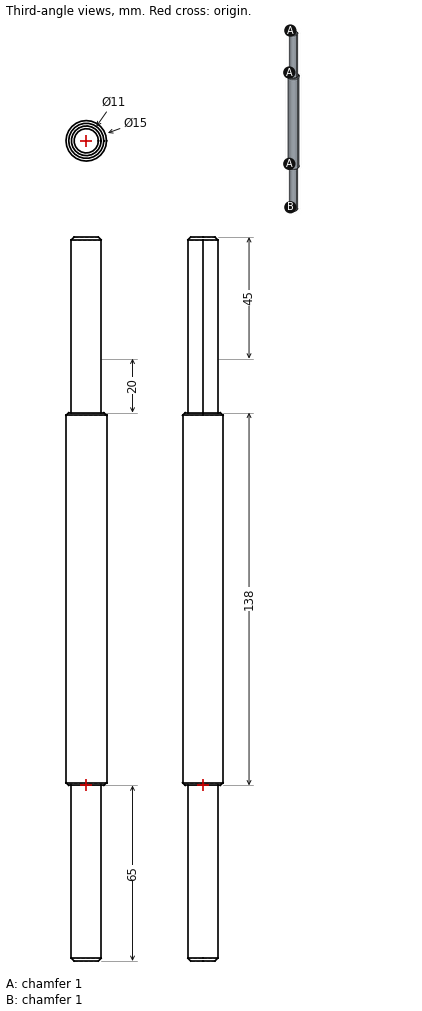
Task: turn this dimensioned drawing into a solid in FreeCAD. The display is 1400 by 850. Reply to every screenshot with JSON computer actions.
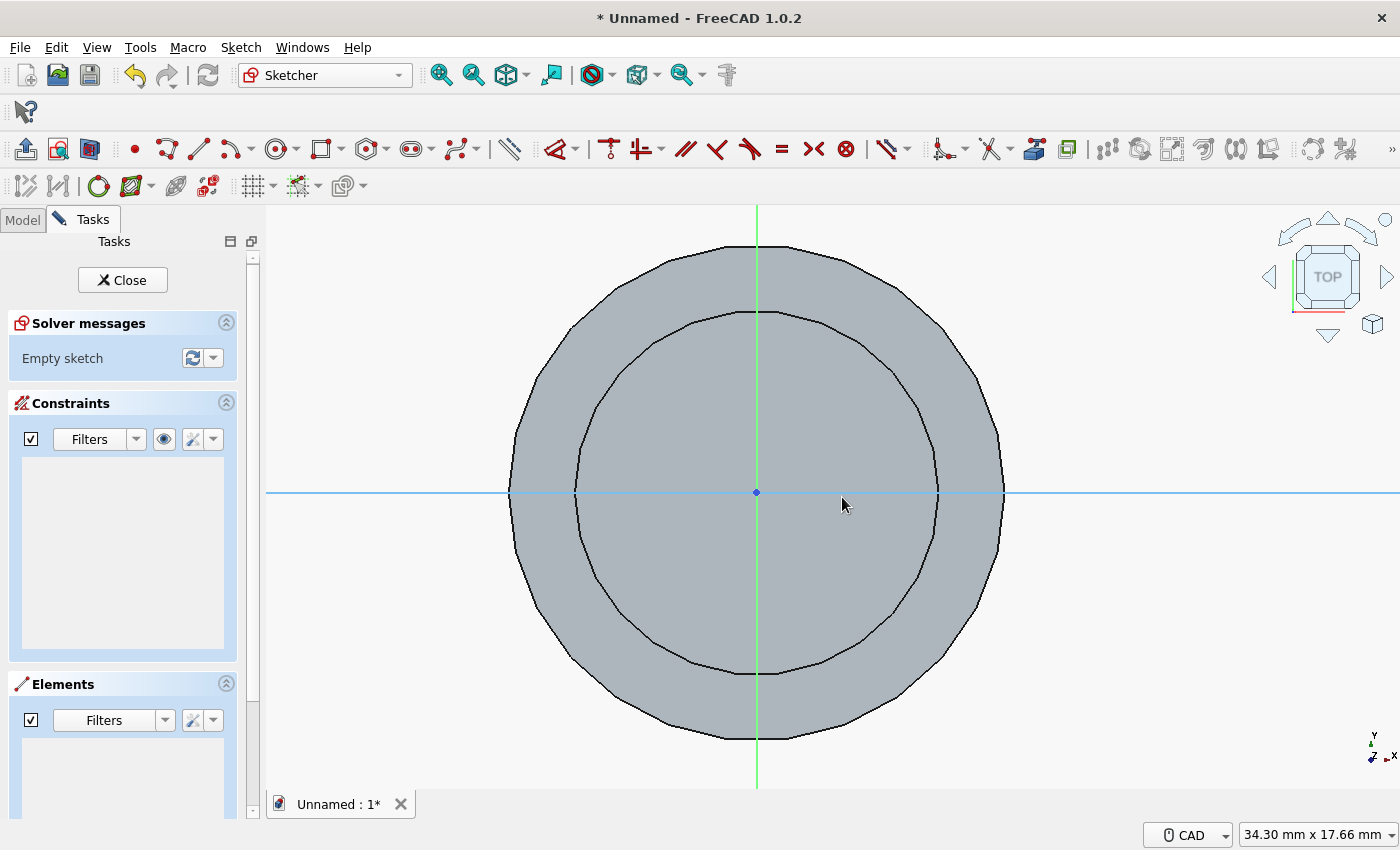
{"action": "left_click", "coordinate": [276, 150]}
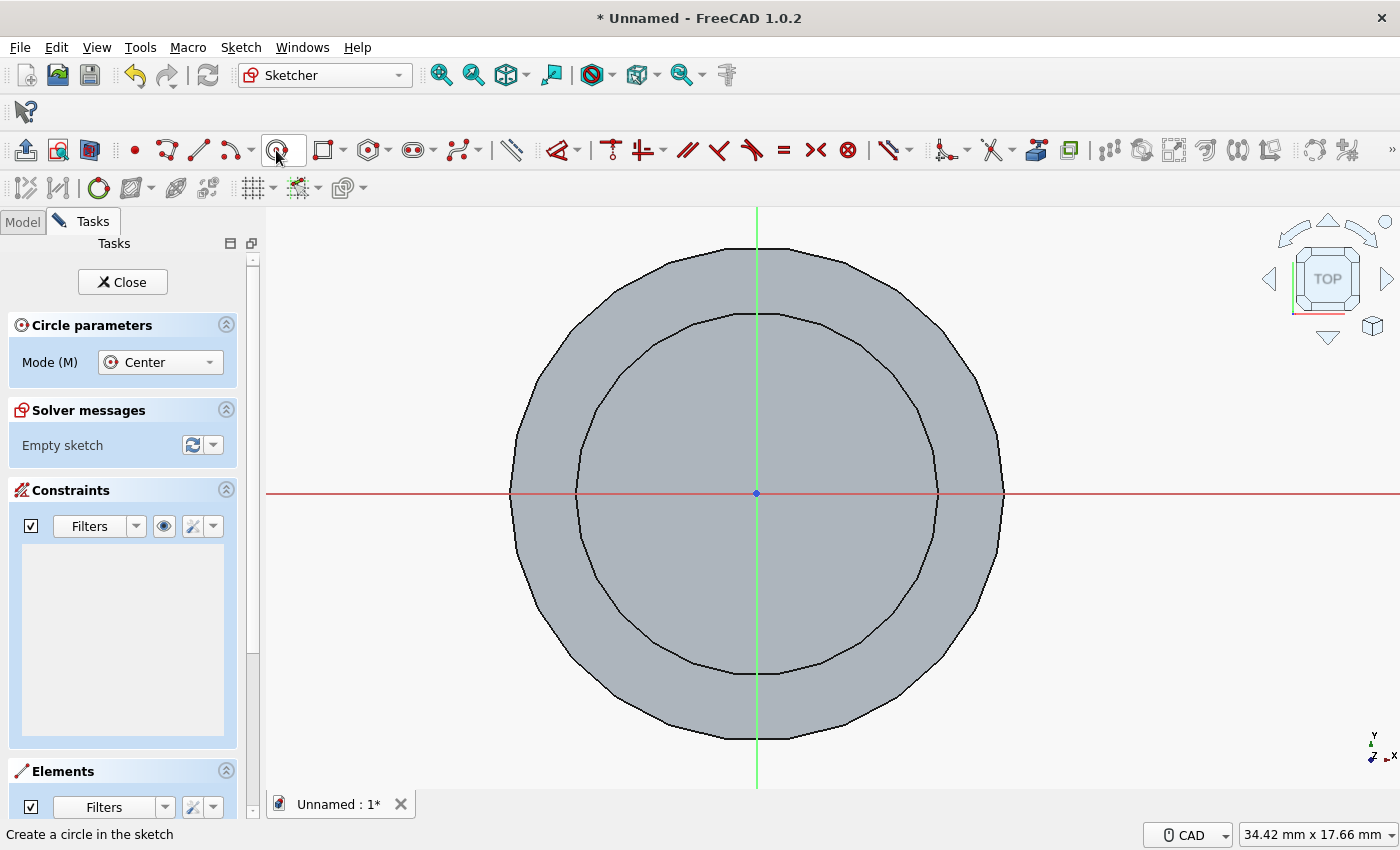
{"action": "left_click", "coordinate": [757, 494]}
{"action": "mouse_move", "coordinate": [885, 366]}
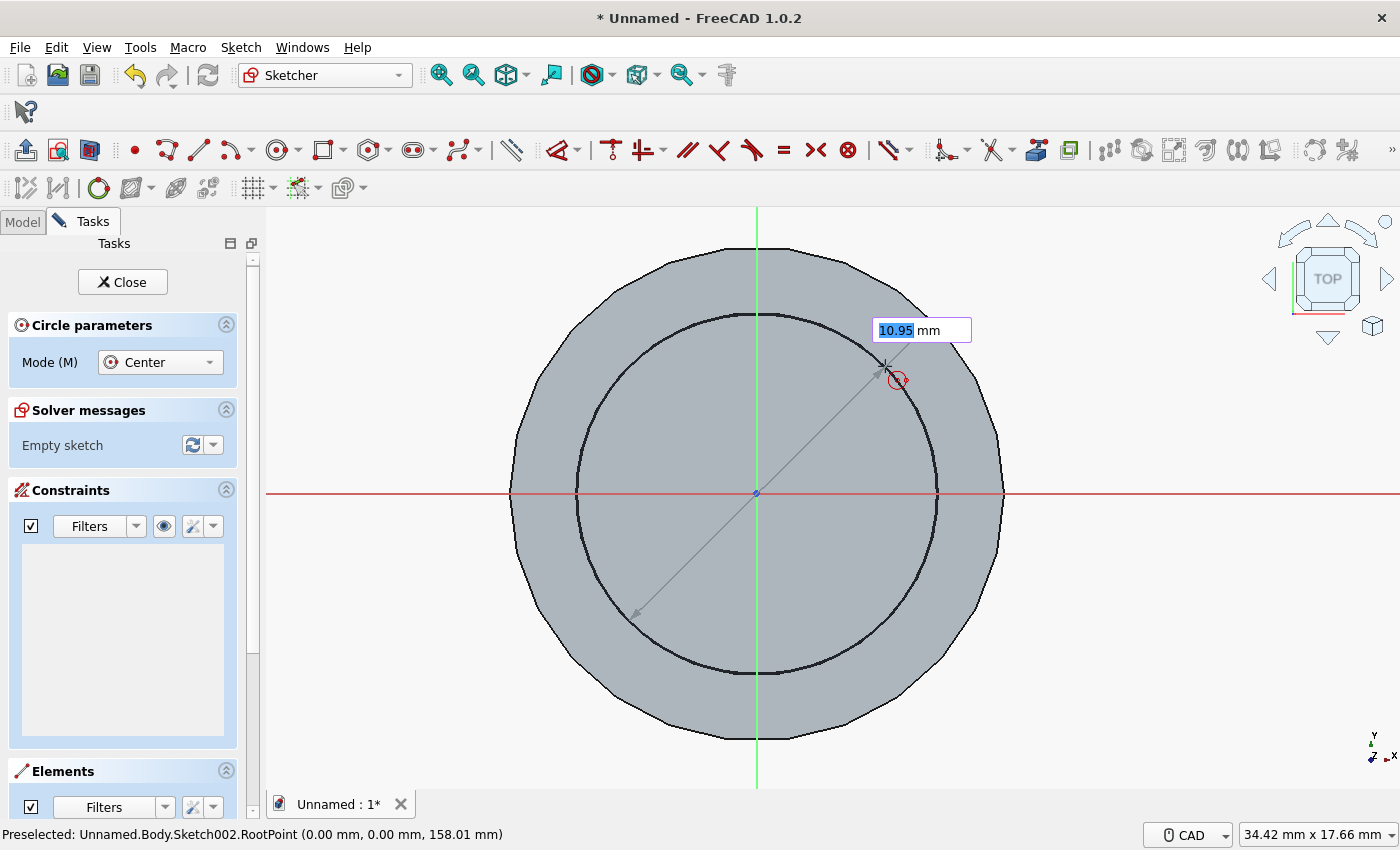
{"action": "type", "text": "11"}
{"action": "key", "text": "Return"}
{"action": "key", "text": "Escape"}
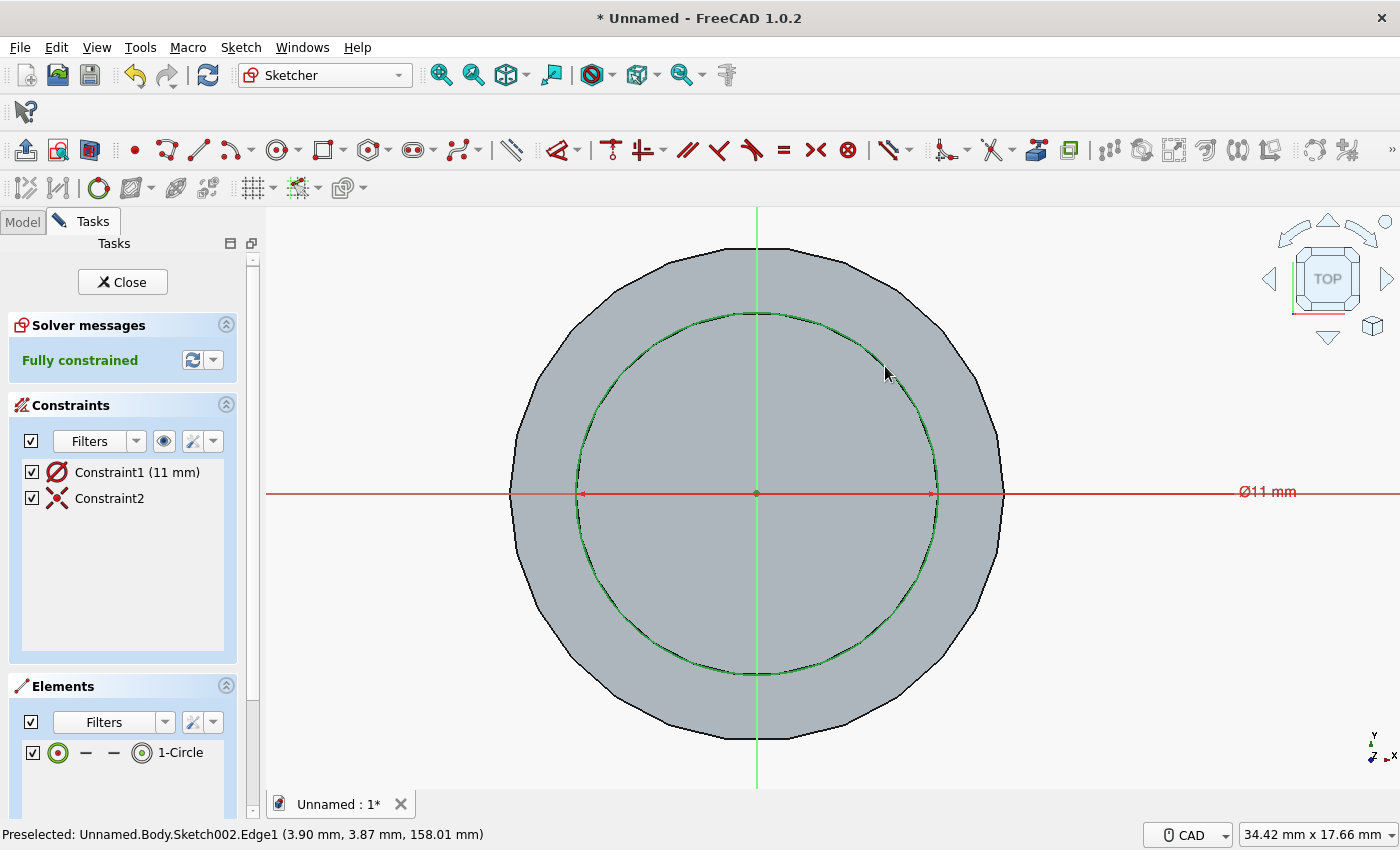
{"action": "left_click", "coordinate": [123, 282]}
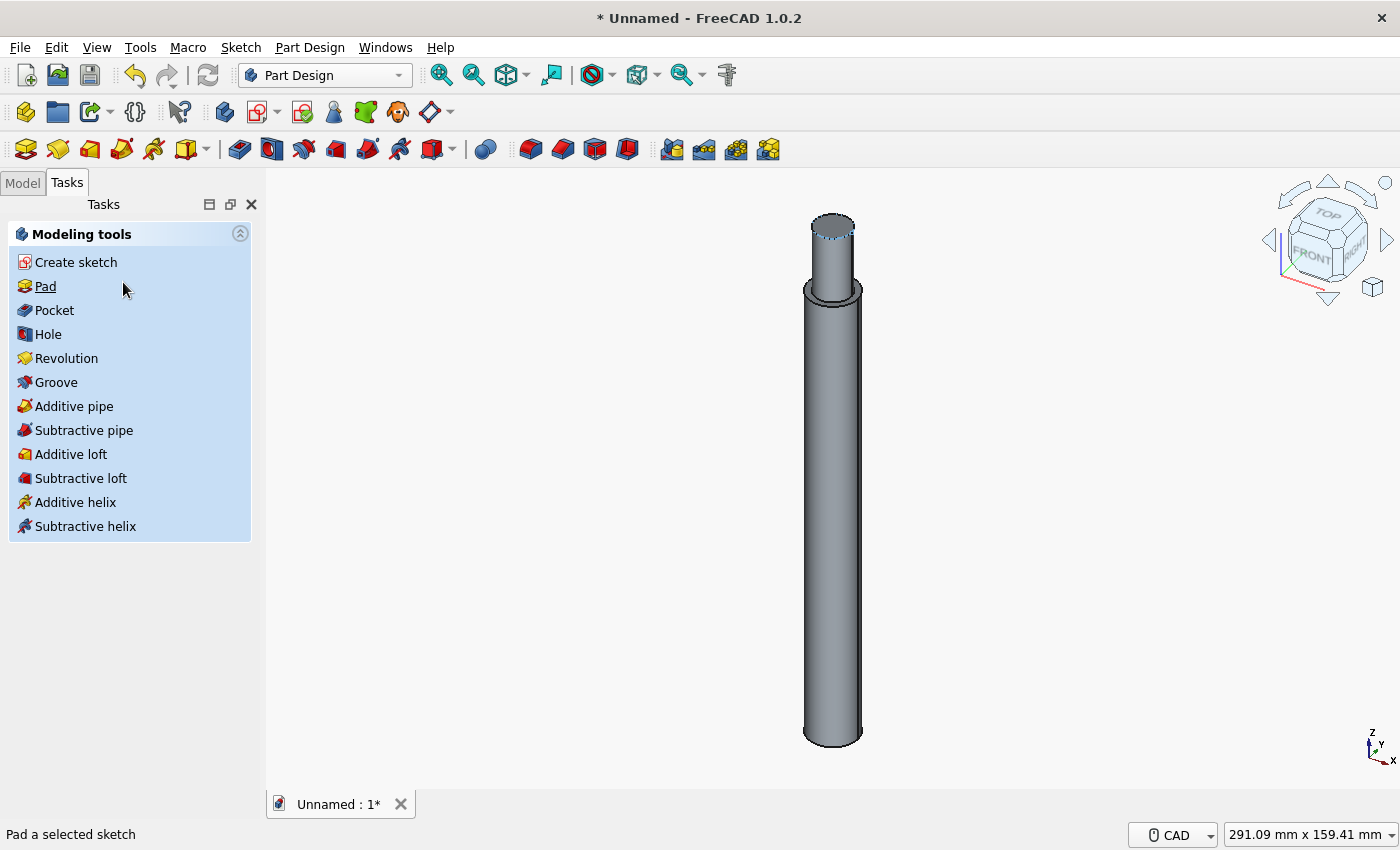
{"action": "left_click", "coordinate": [26, 150]}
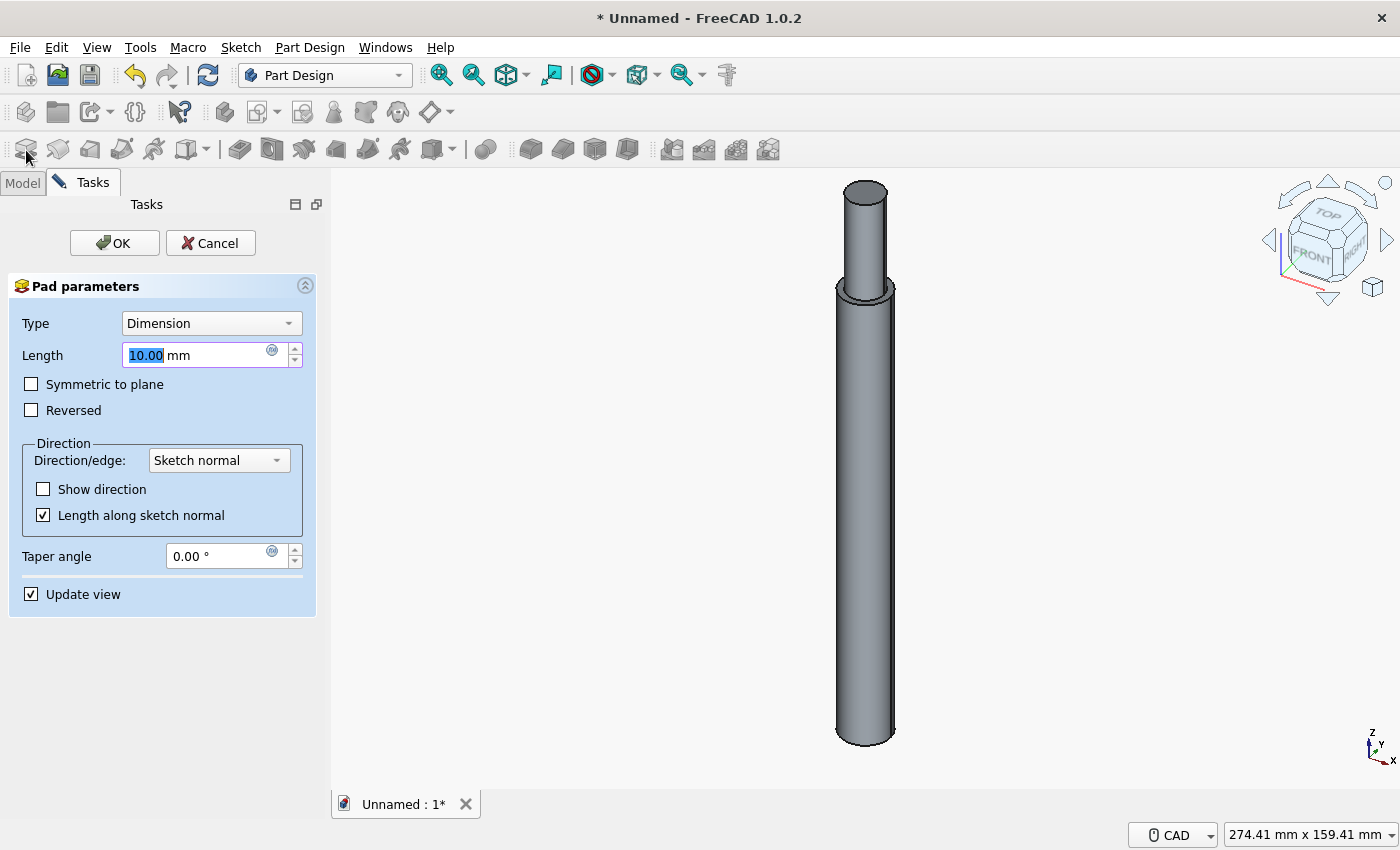
{"action": "type", "text": "45"}
{"action": "key", "text": "Tab"}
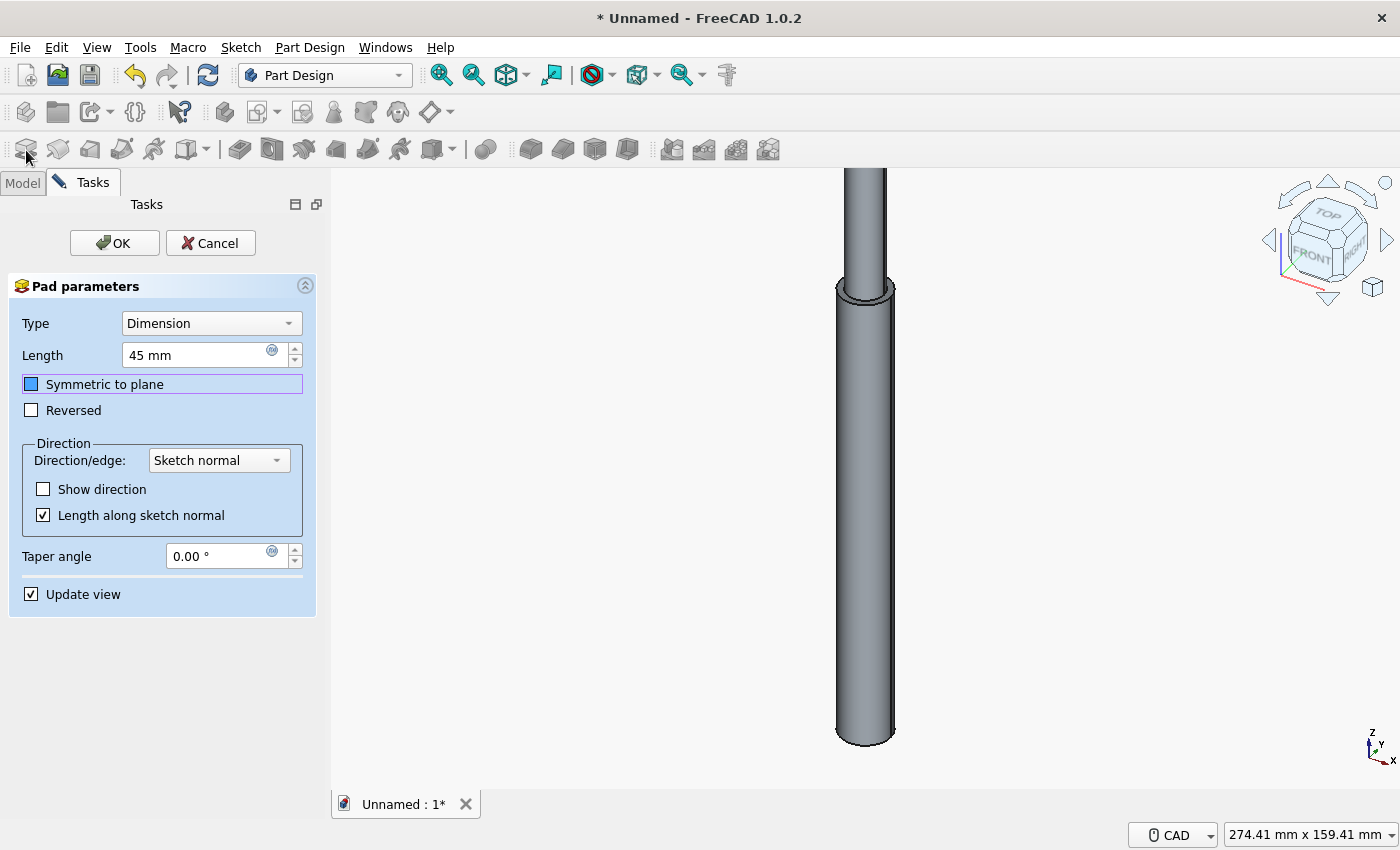
{"action": "left_click", "coordinate": [115, 243]}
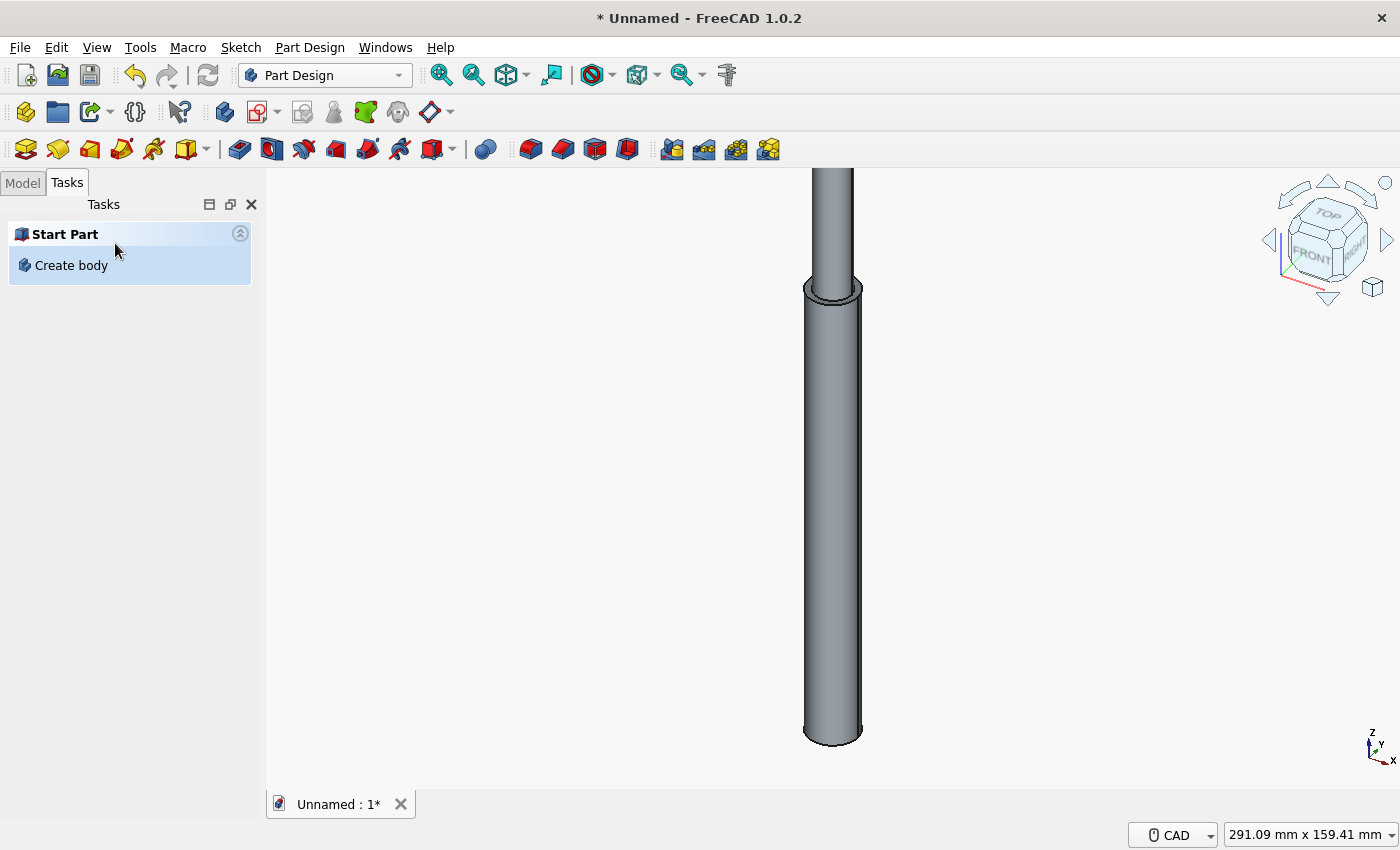
{"action": "key", "text": "v f"}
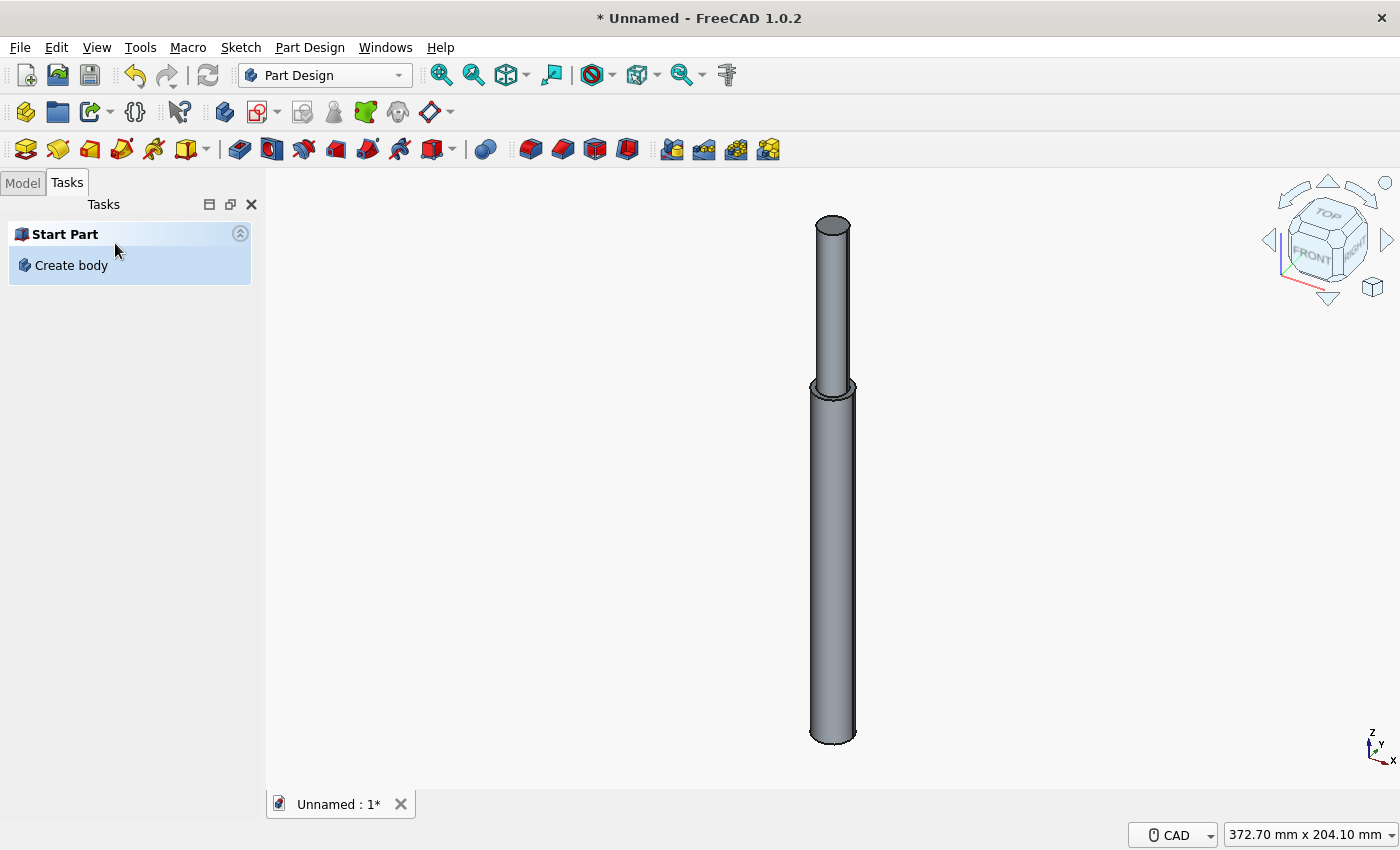
{"action": "left_click", "coordinate": [816, 739]}